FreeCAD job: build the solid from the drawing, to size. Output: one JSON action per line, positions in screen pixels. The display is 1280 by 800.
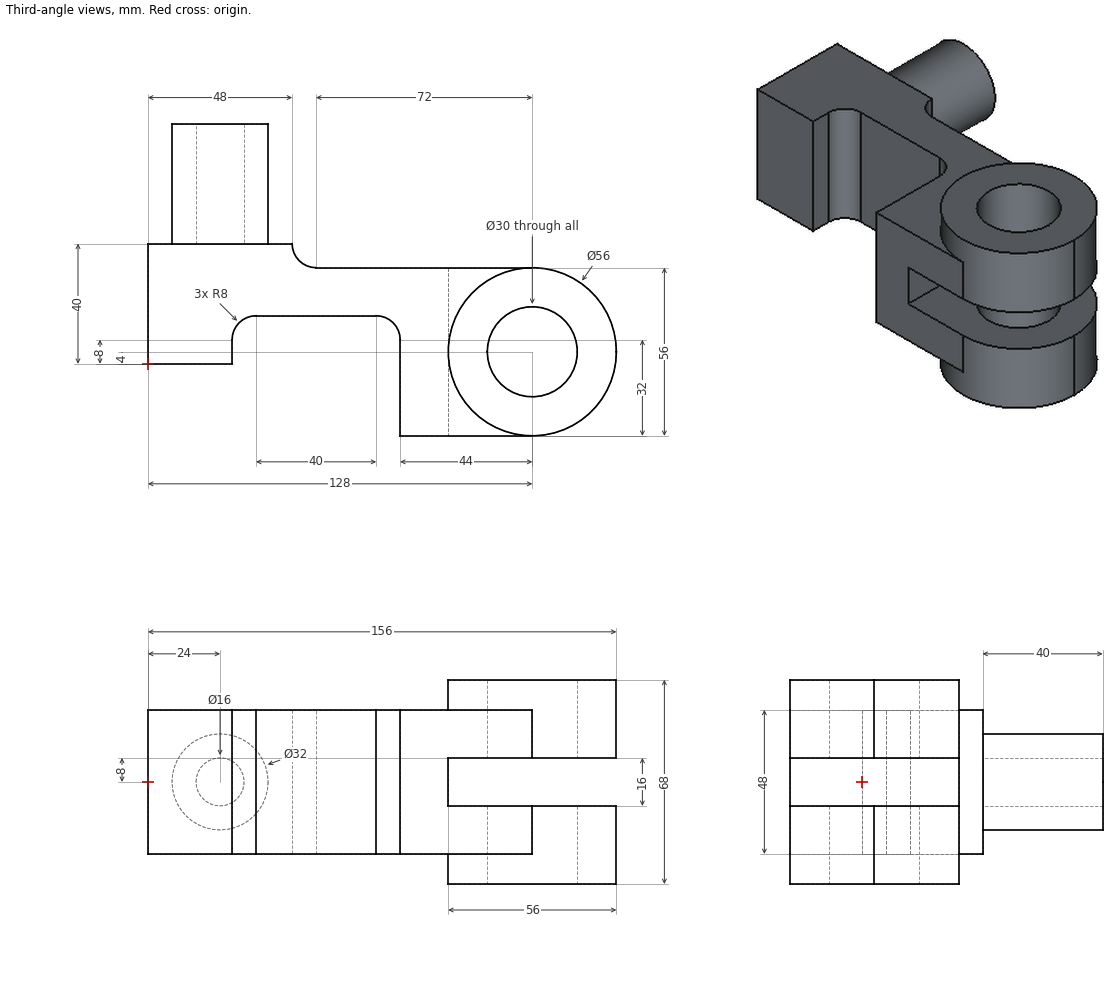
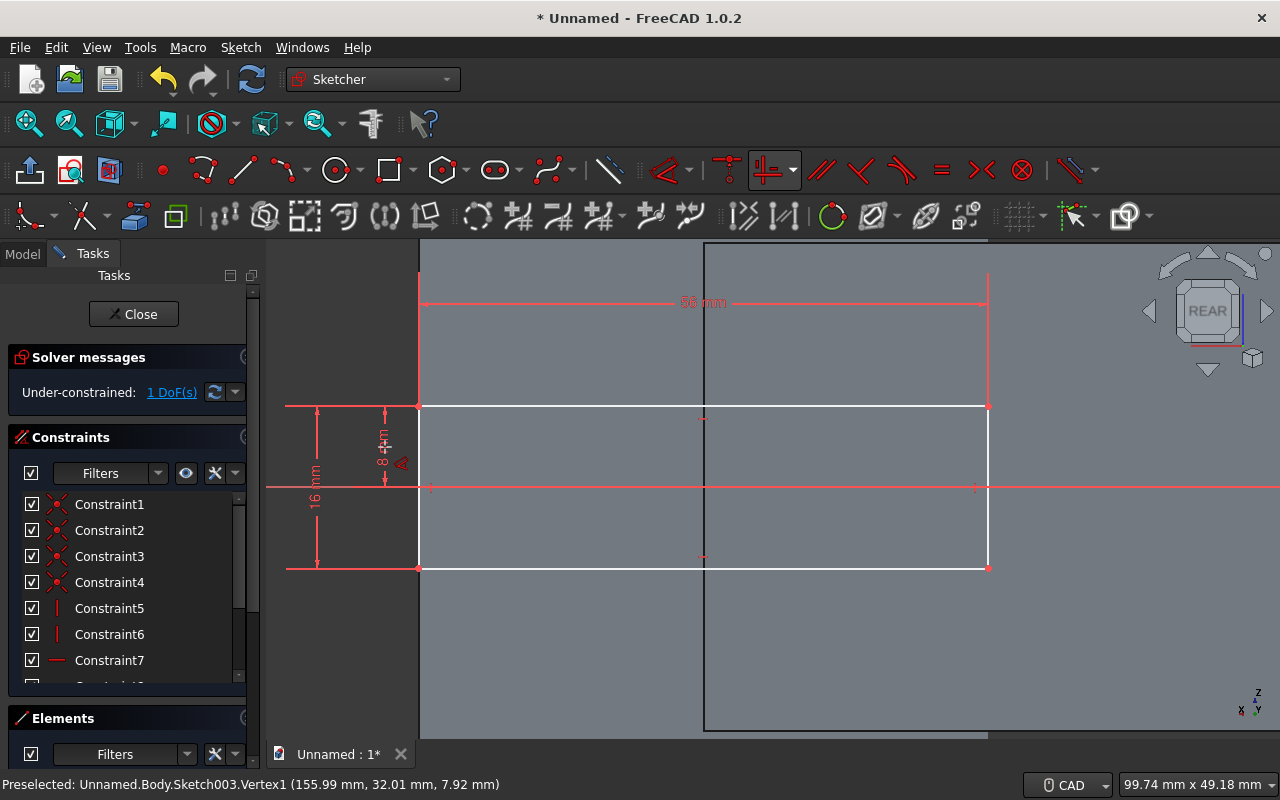
{"action": "left_click", "coordinate": [419, 406]}
{"action": "left_click", "coordinate": [767, 372]}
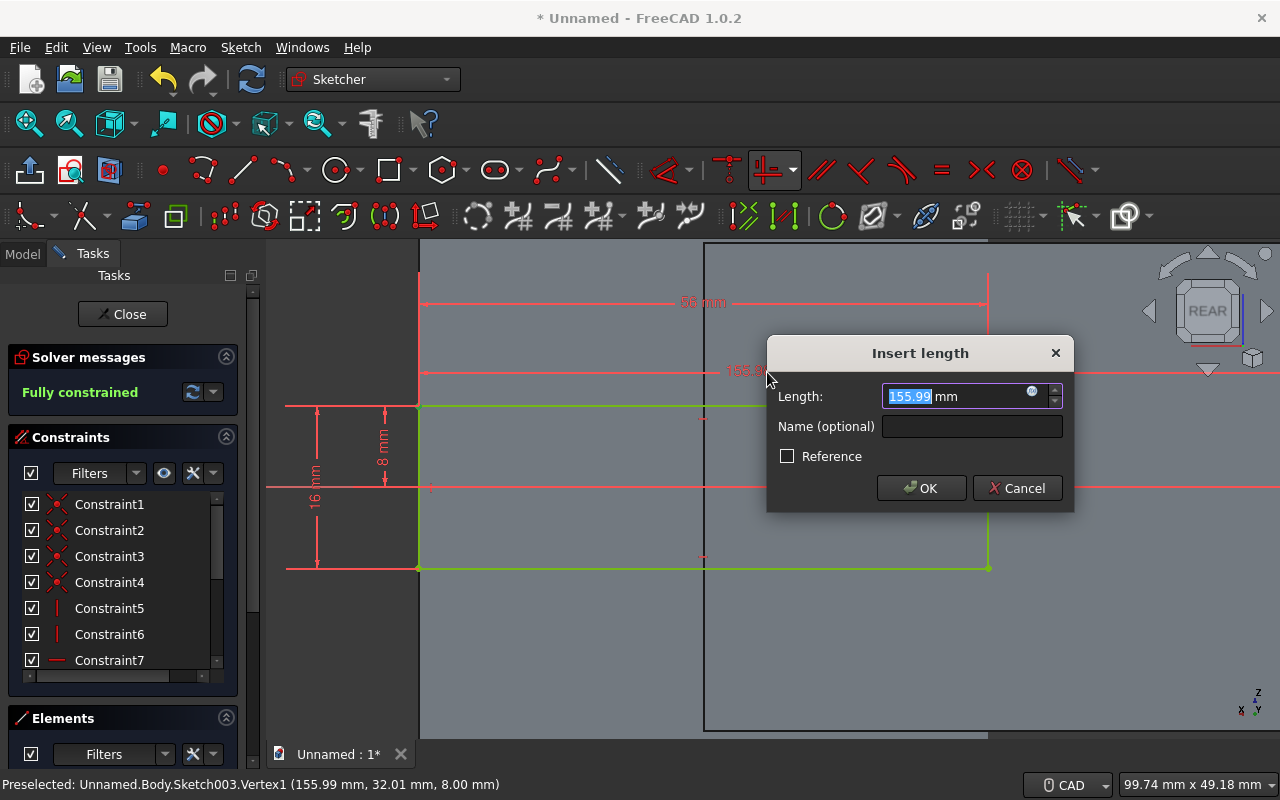
{"action": "type", "text": "156"}
{"action": "key", "text": "Return"}
{"action": "key", "text": "Escape"}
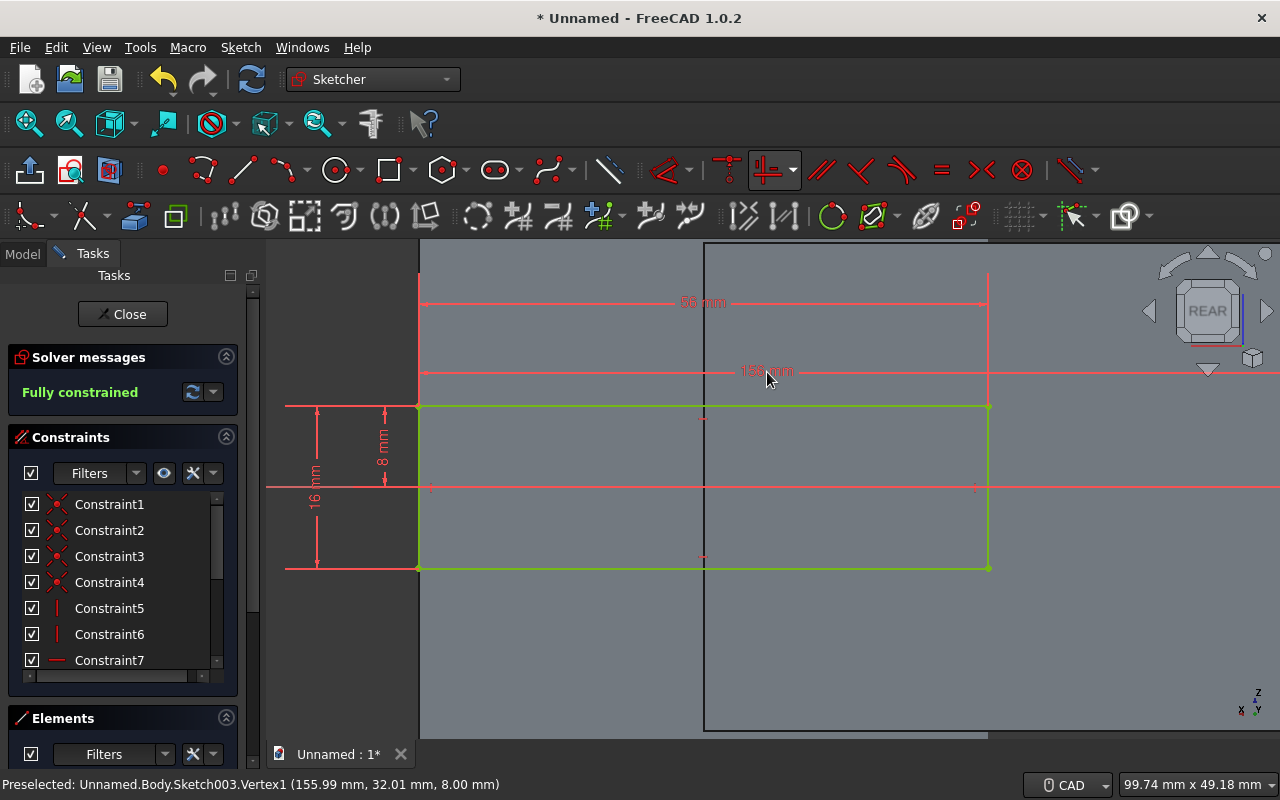
{"action": "left_click", "coordinate": [123, 314]}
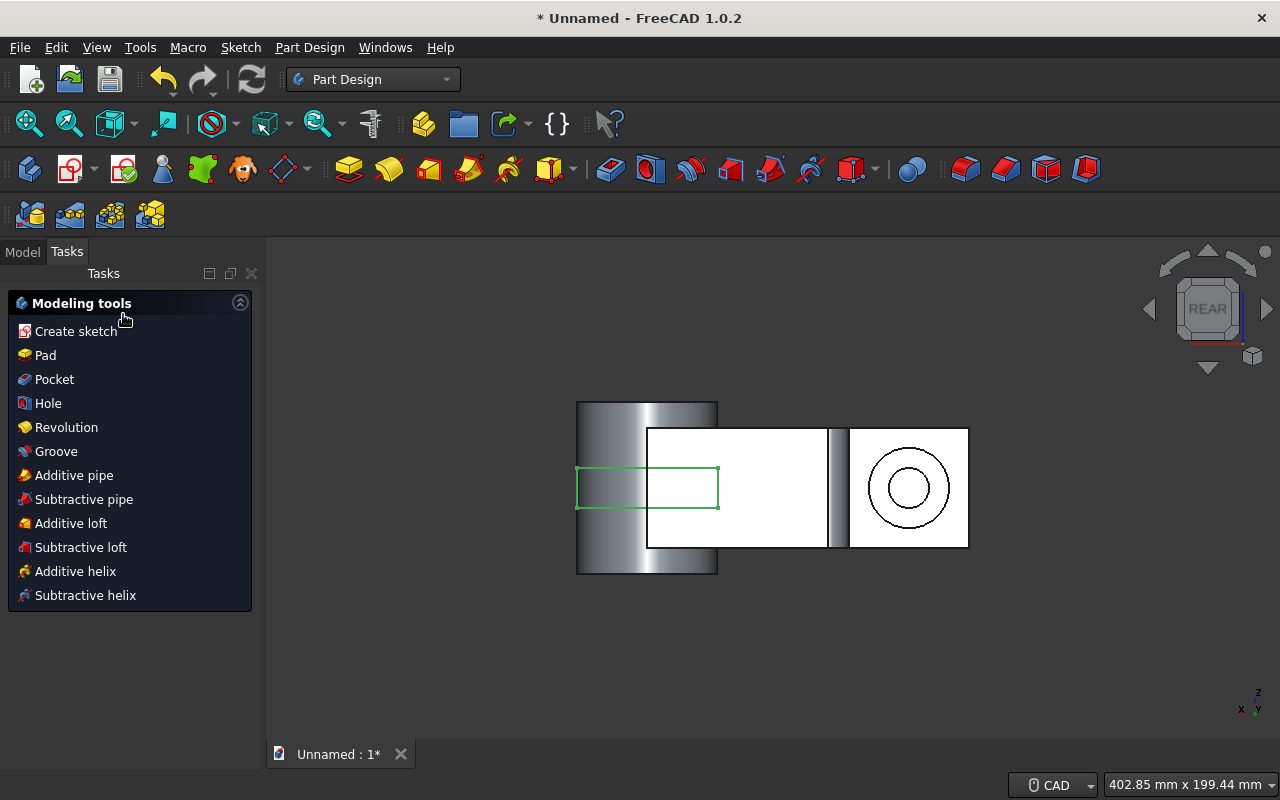
{"action": "left_click", "coordinate": [612, 170]}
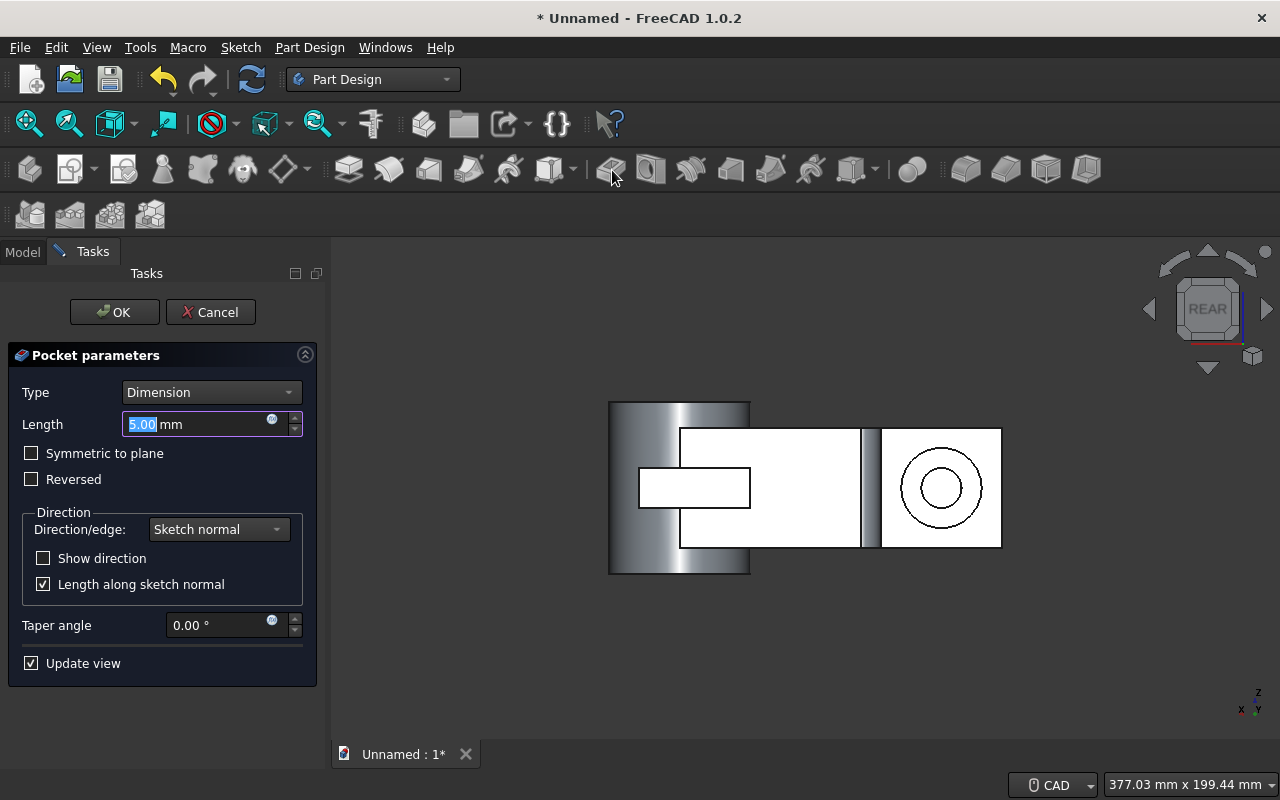
{"action": "left_click", "coordinate": [212, 392]}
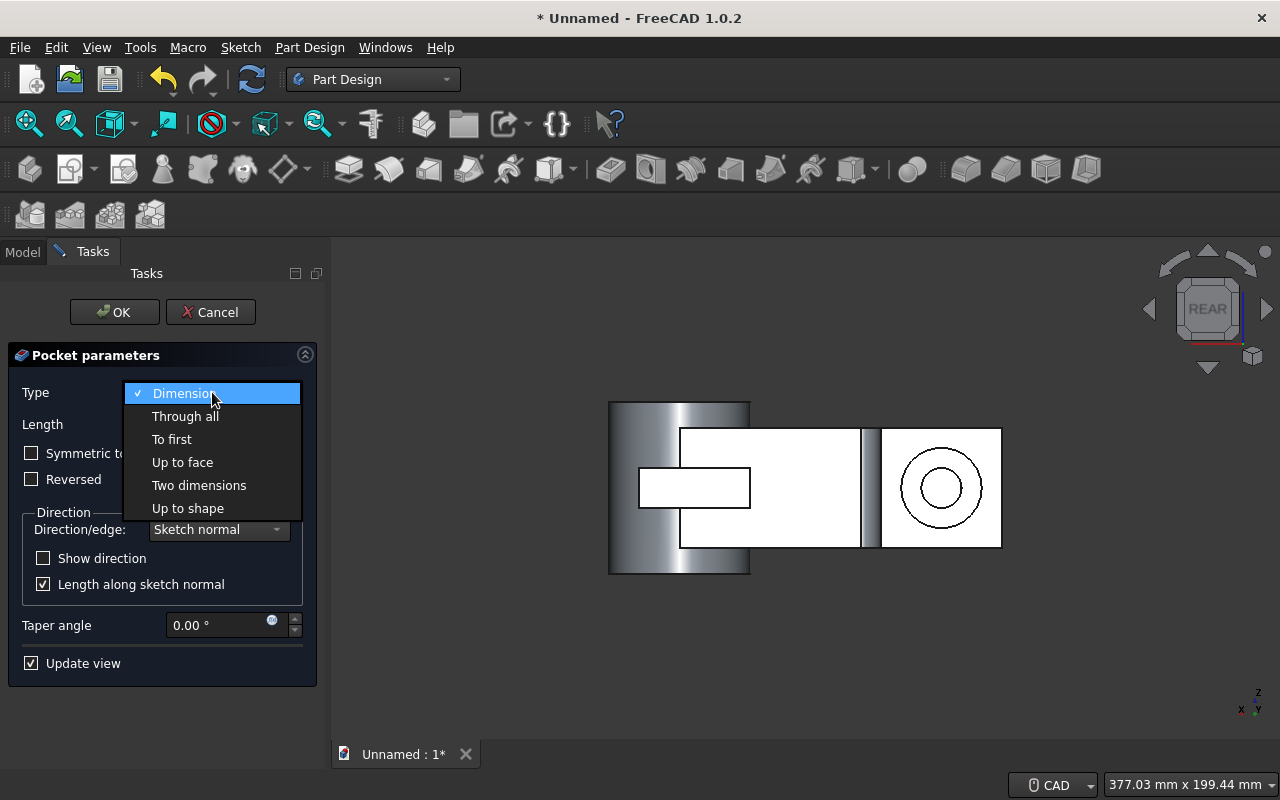
{"action": "left_click", "coordinate": [212, 416]}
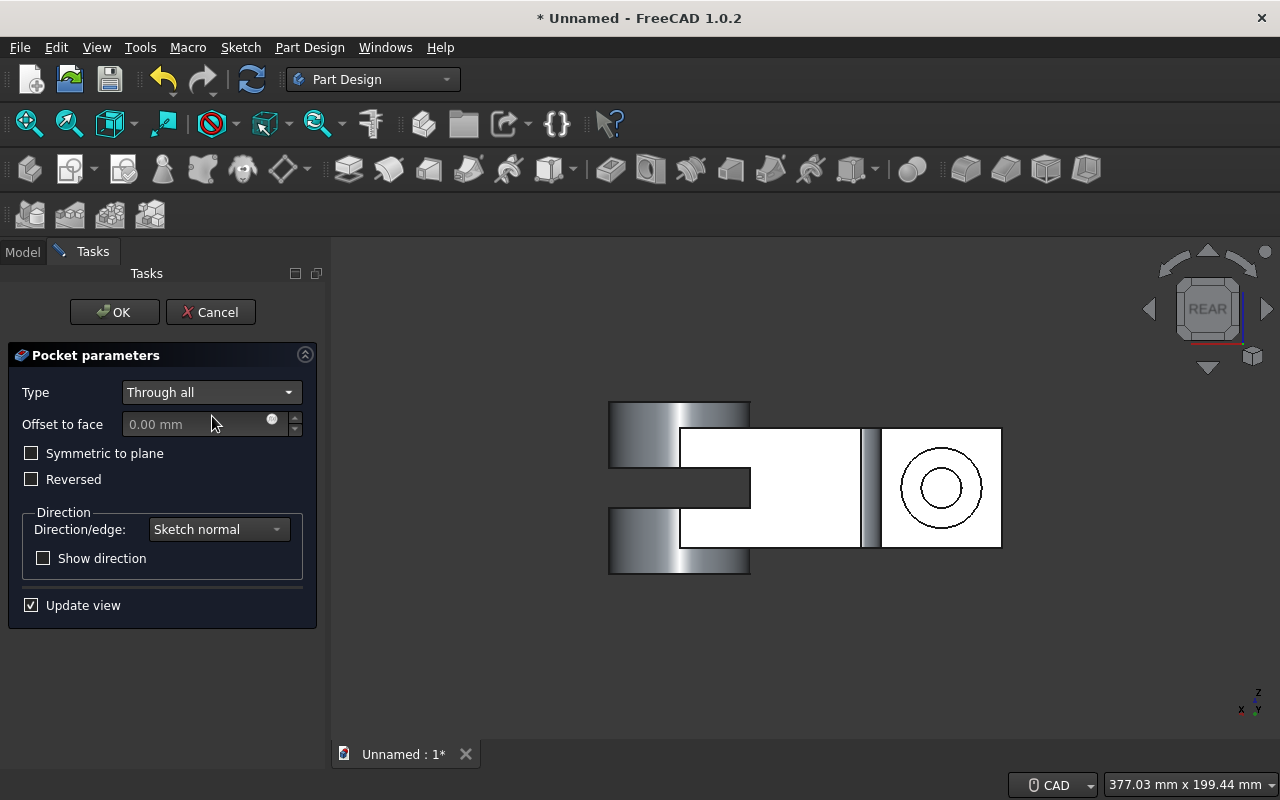
{"action": "left_click", "coordinate": [115, 312]}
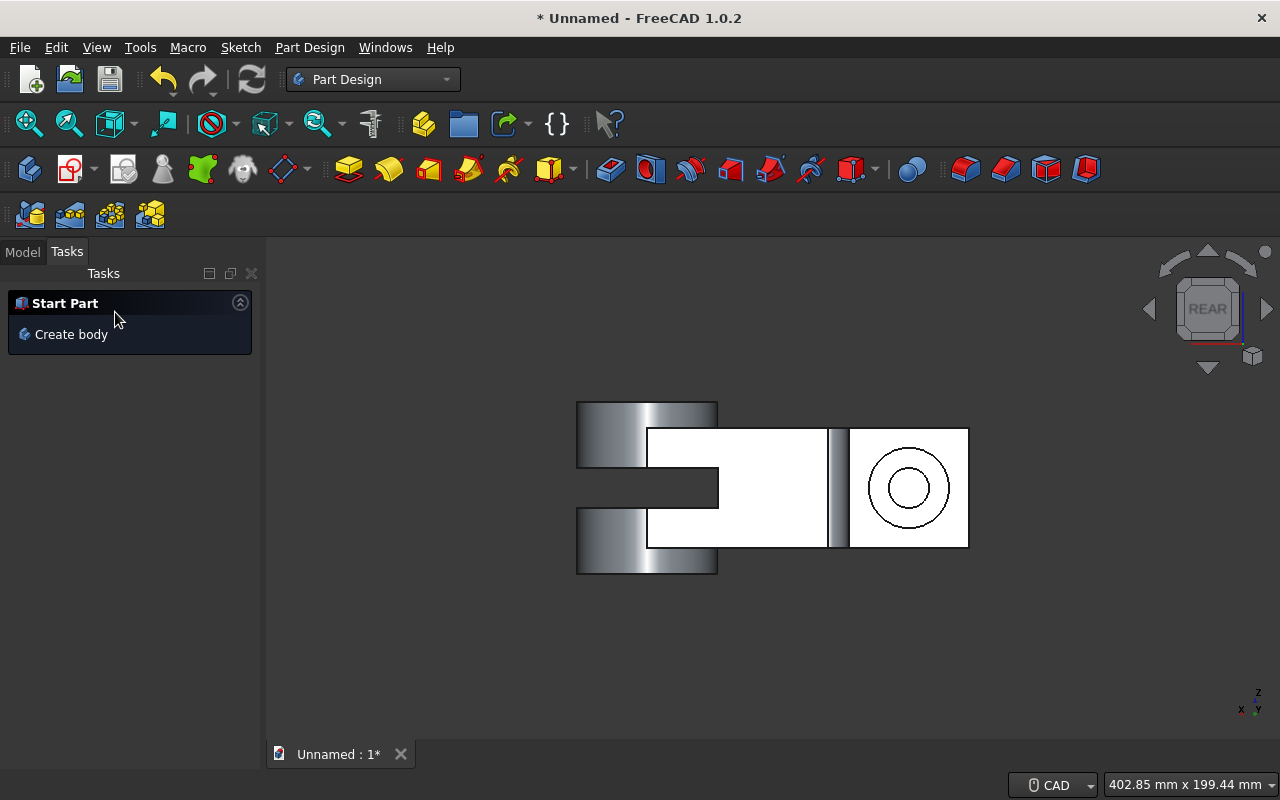
{"action": "key", "text": "v f"}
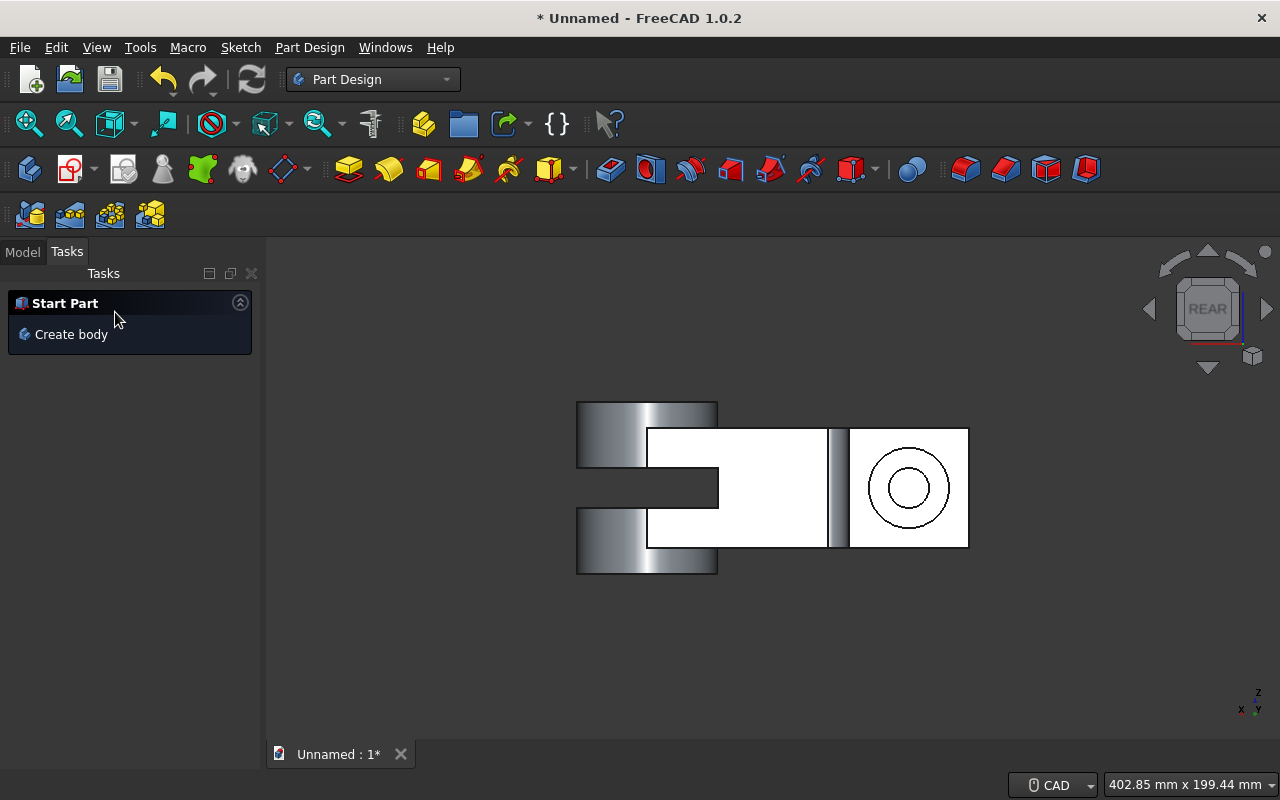
{"action": "key", "text": "0"}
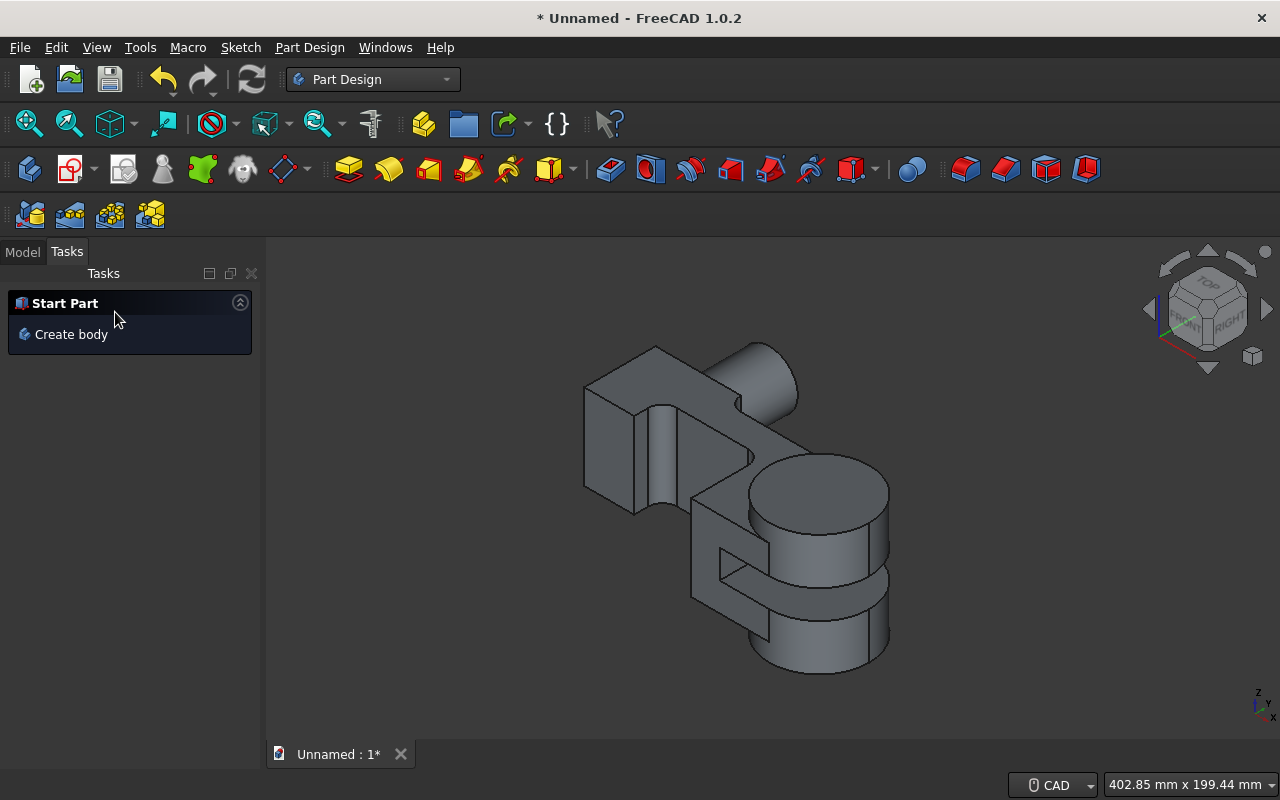
{"action": "left_click", "coordinate": [819, 493]}